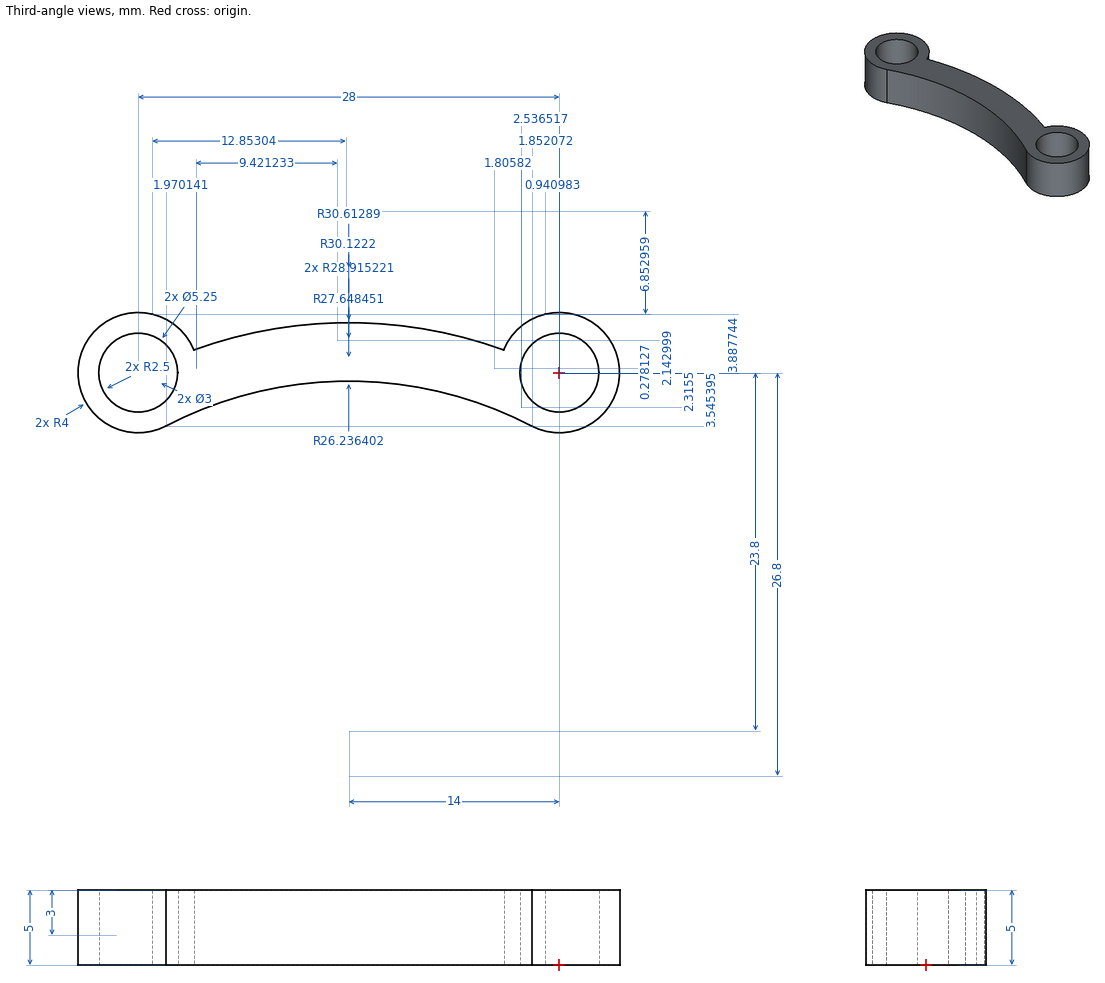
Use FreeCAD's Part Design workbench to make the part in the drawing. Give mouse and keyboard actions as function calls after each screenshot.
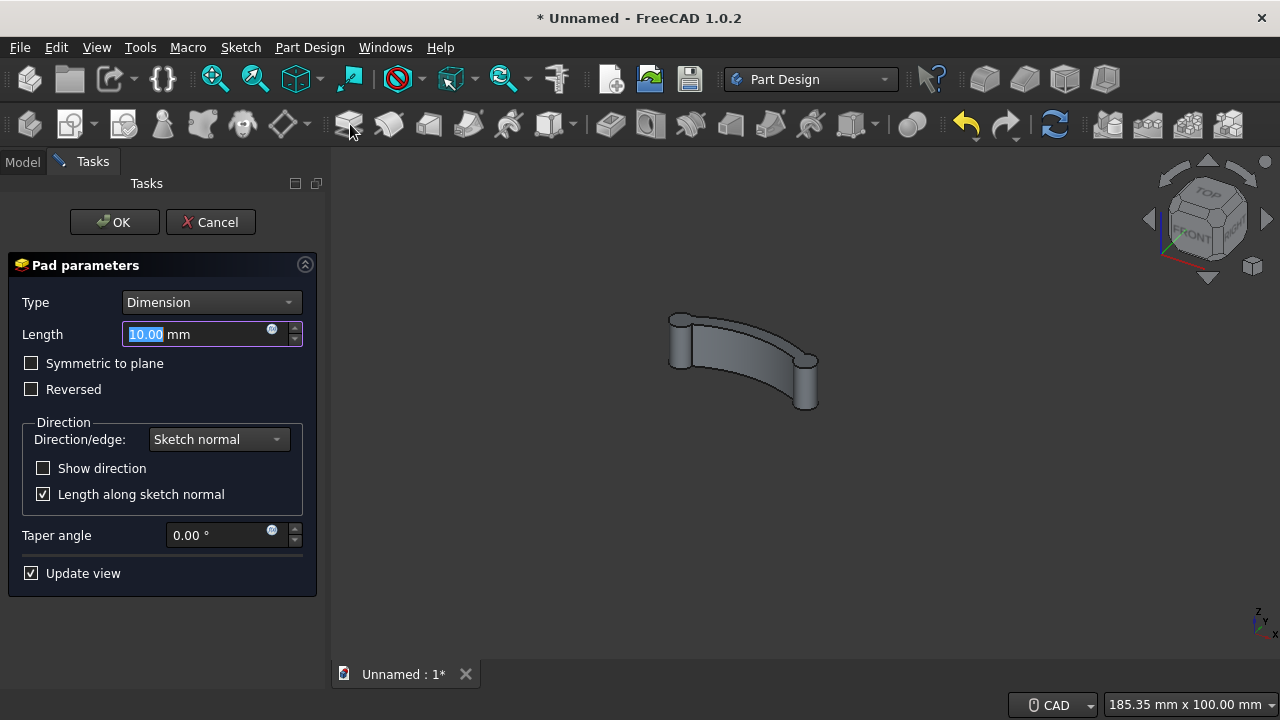
text(5)
key(Tab)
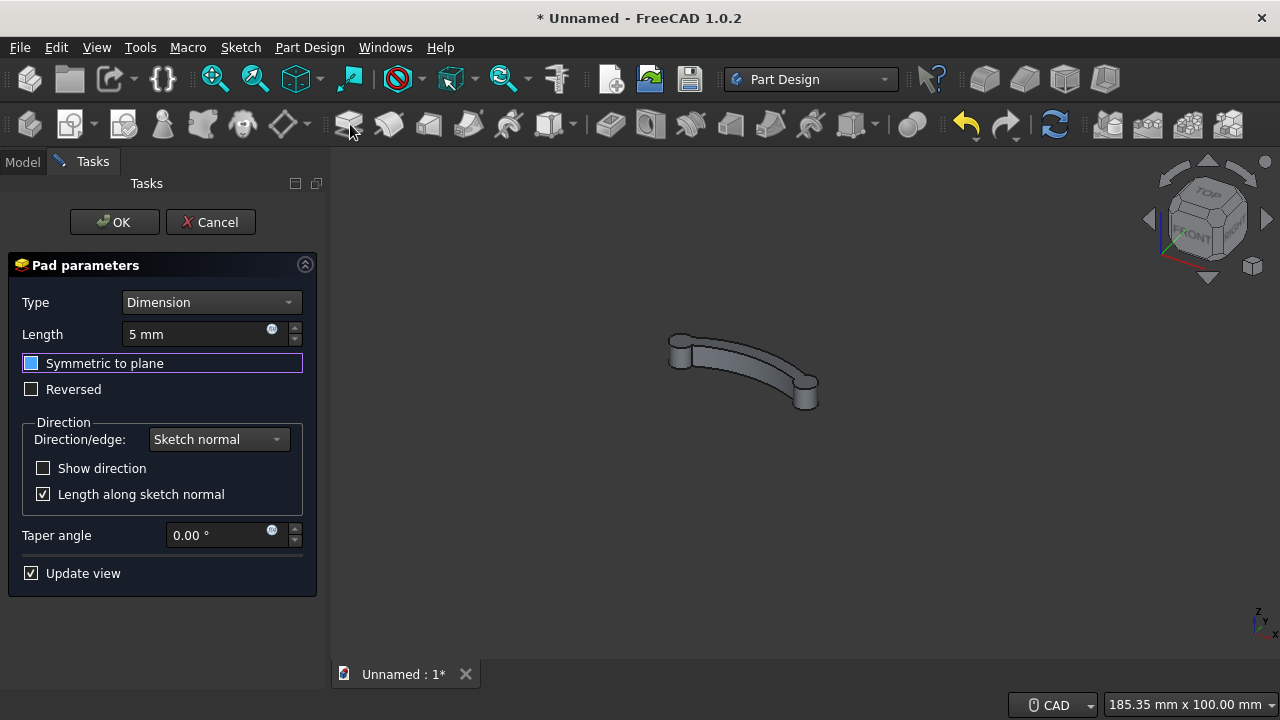
click(115, 222)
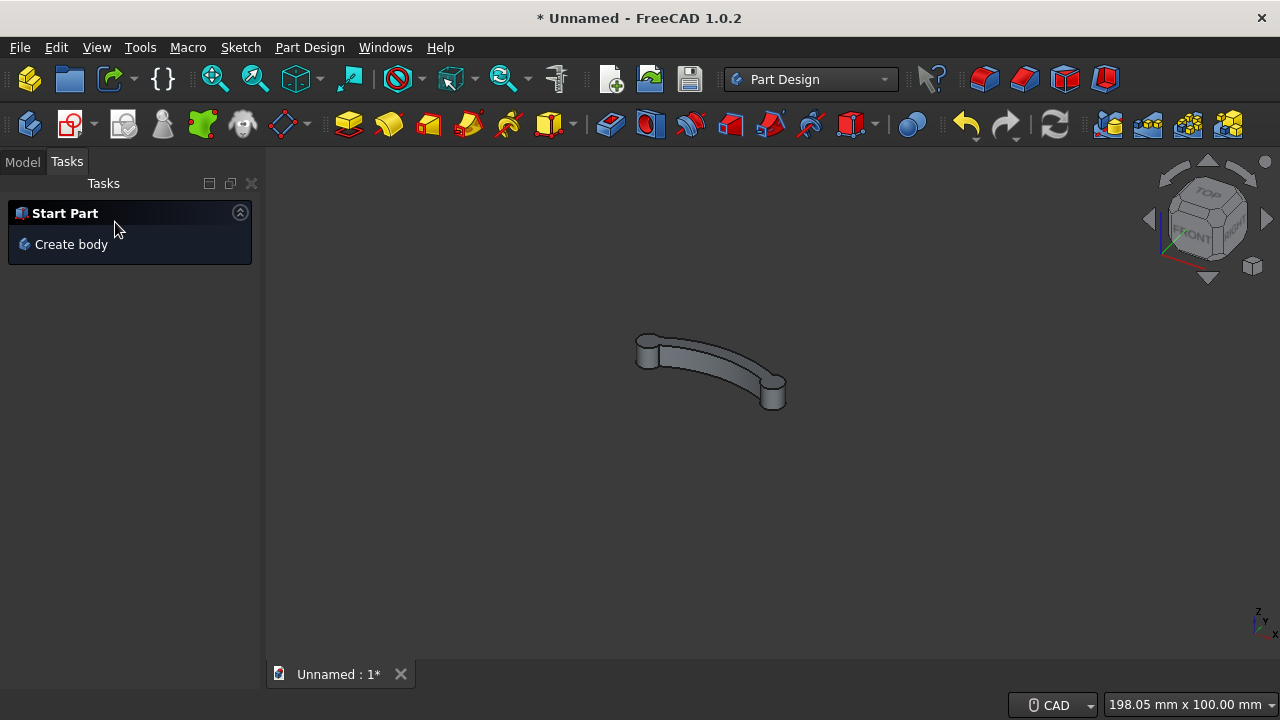
click(216, 80)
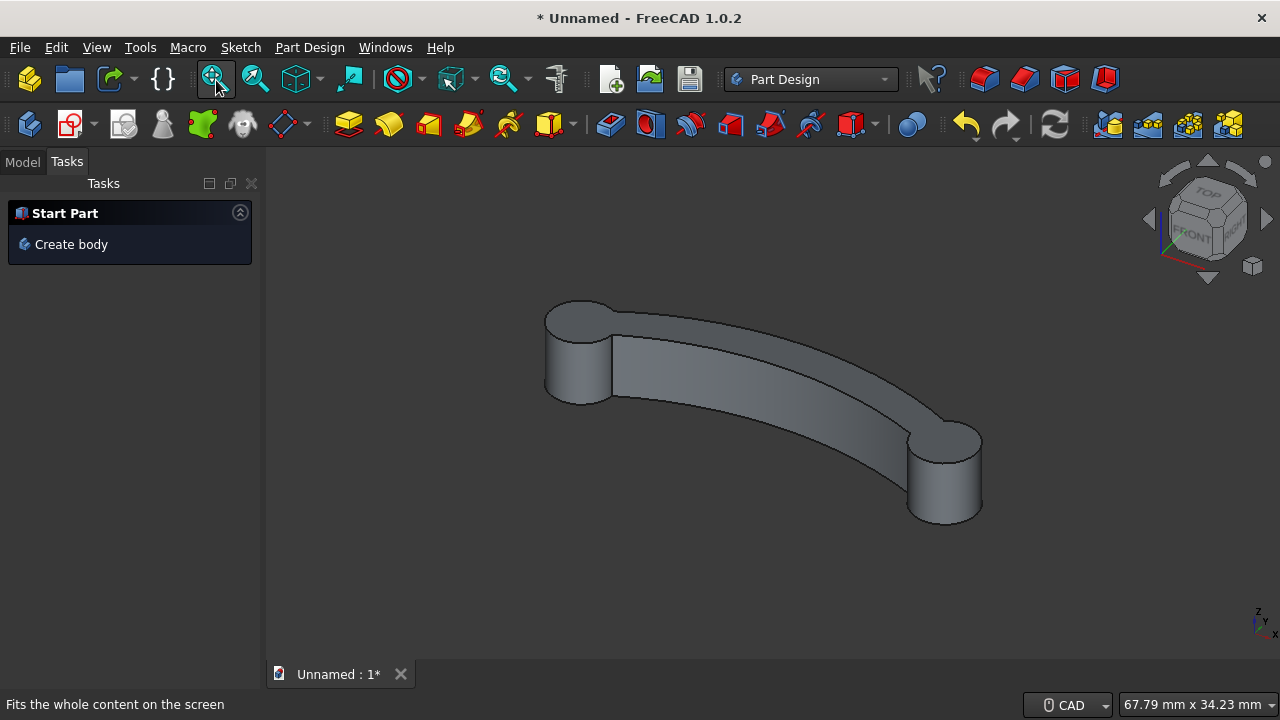
click(582, 319)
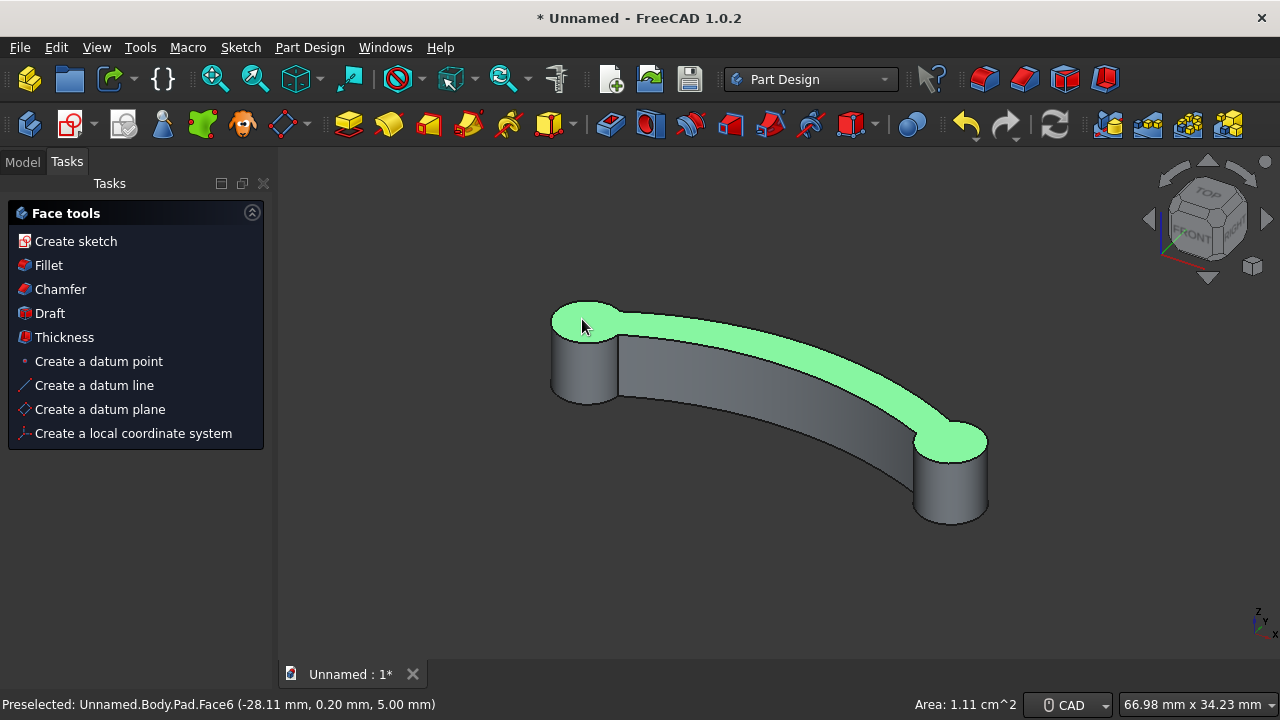
click(70, 124)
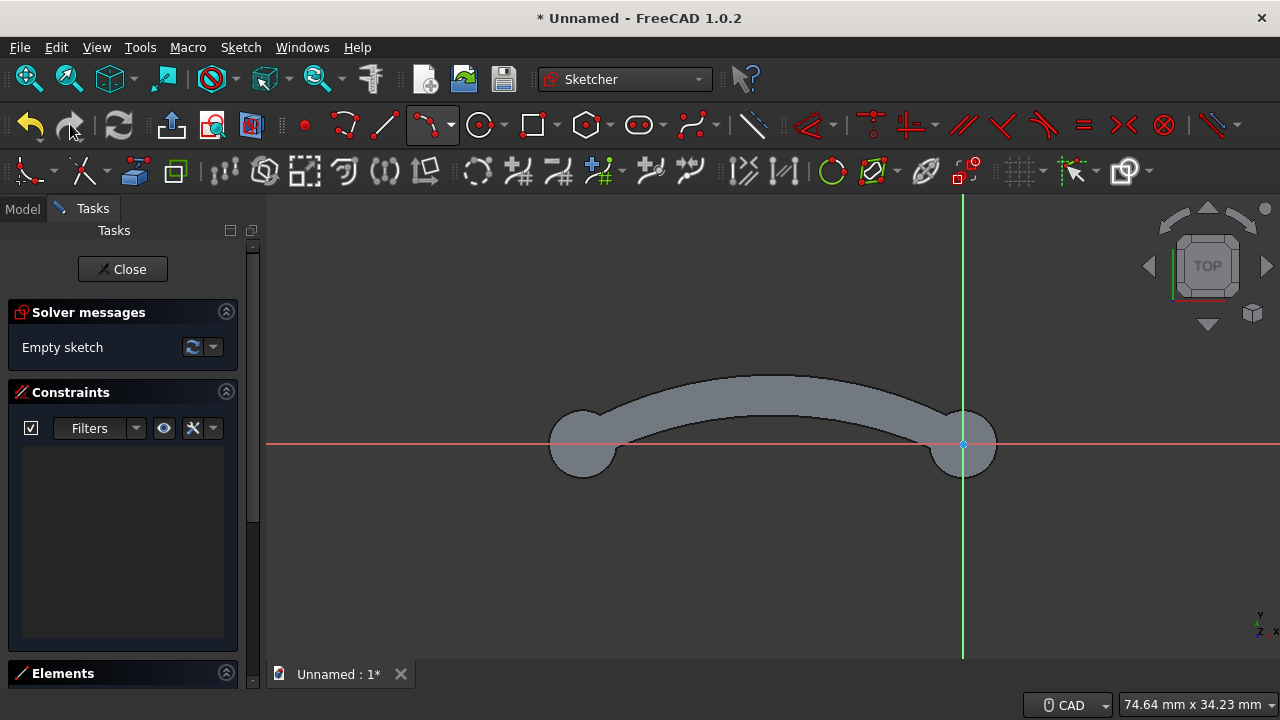
scroll(912, 480, up, 2)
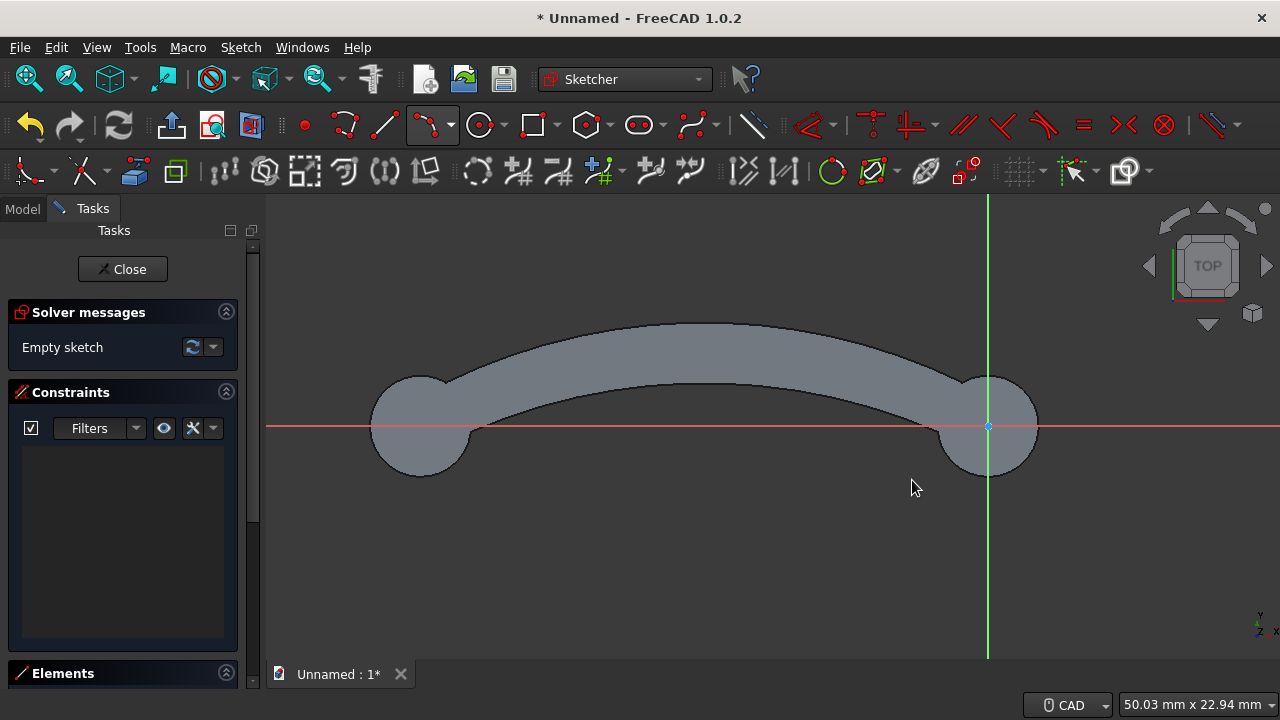
click(480, 126)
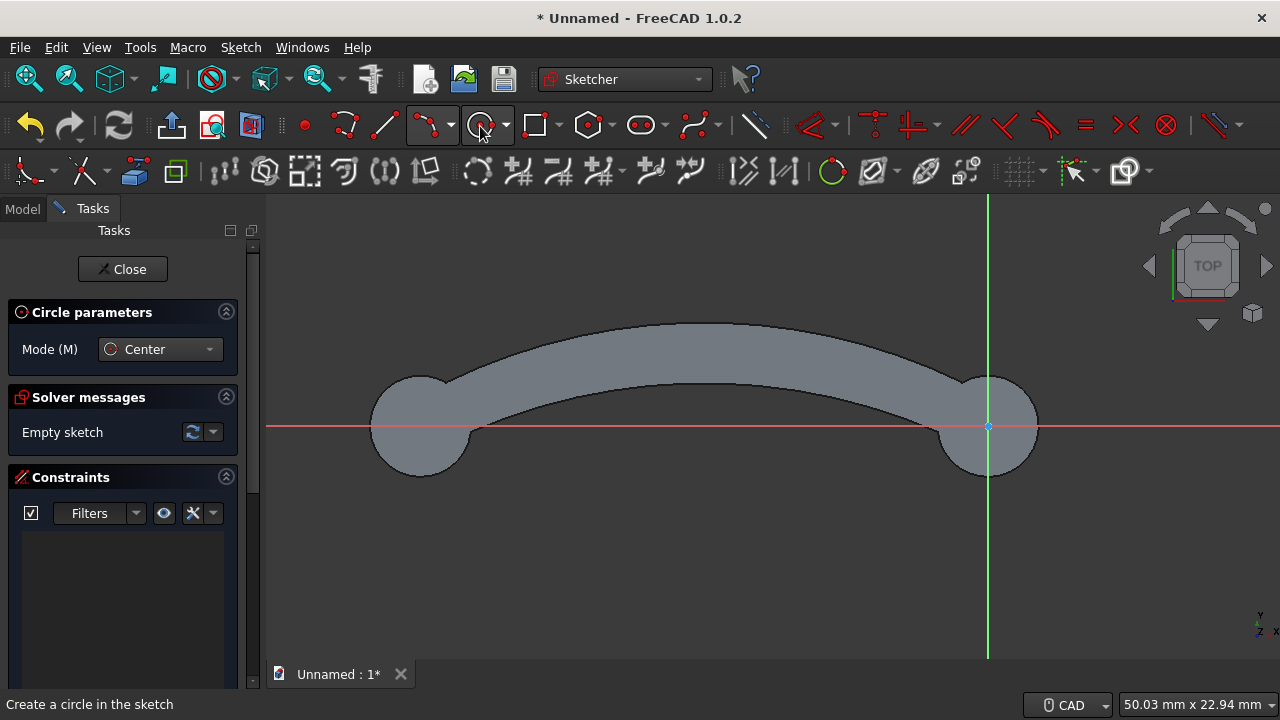
click(421, 426)
click(442, 405)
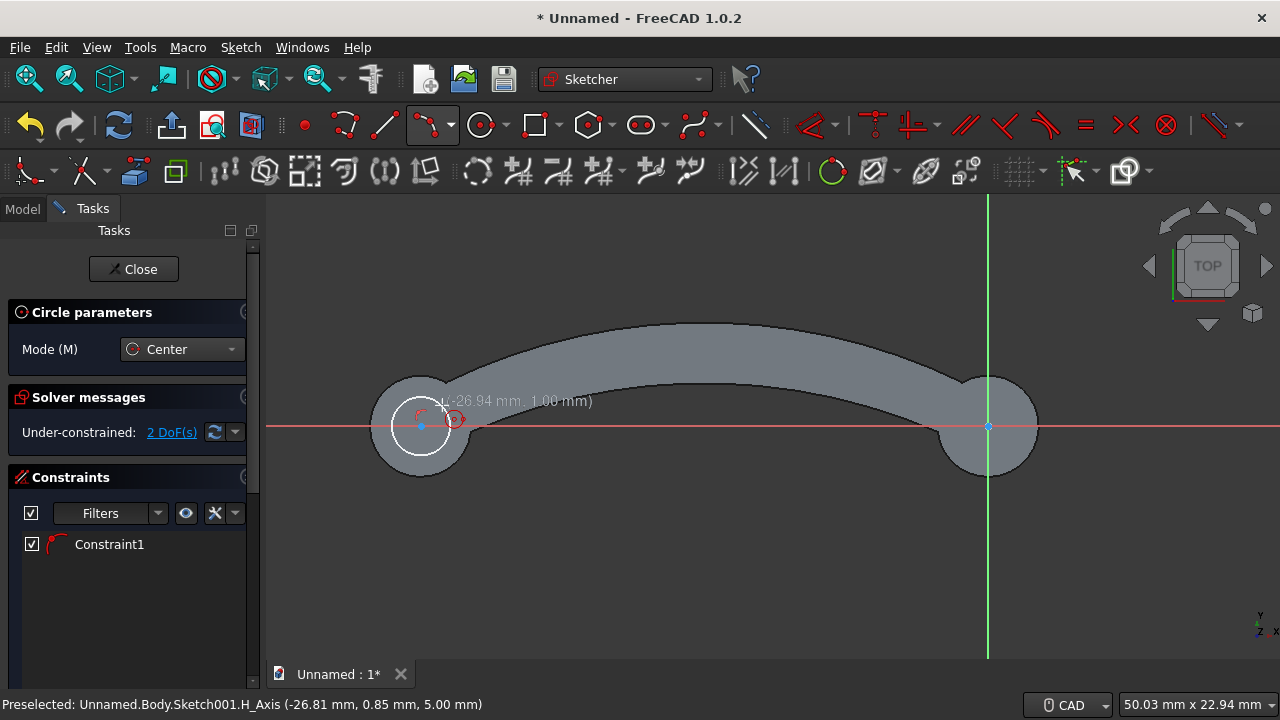
click(988, 426)
click(1010, 405)
key(Escape)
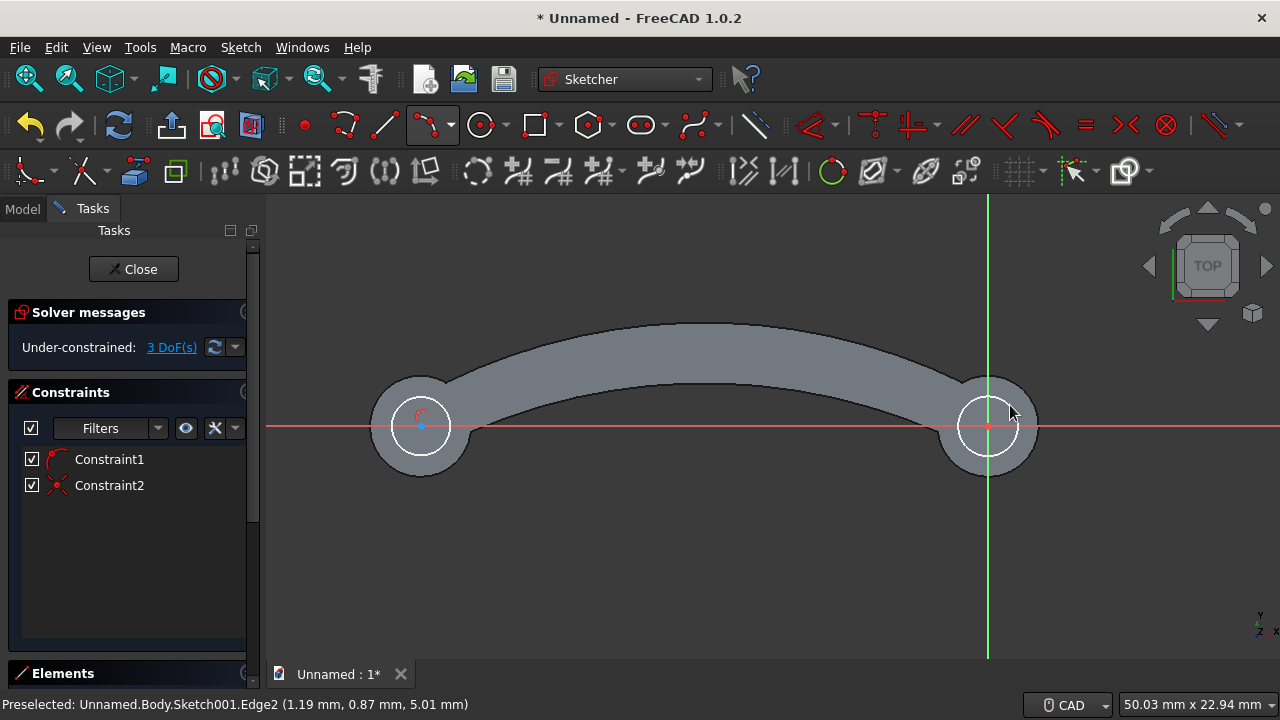
click(442, 406)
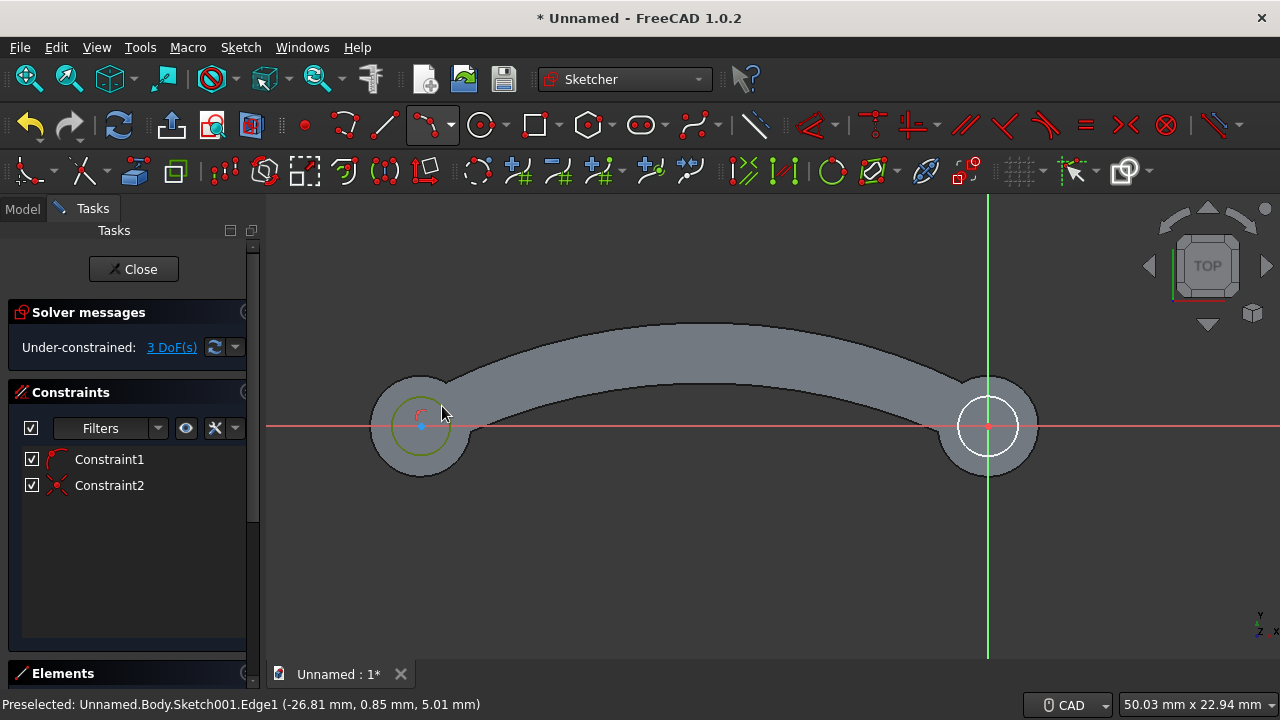
click(1009, 405)